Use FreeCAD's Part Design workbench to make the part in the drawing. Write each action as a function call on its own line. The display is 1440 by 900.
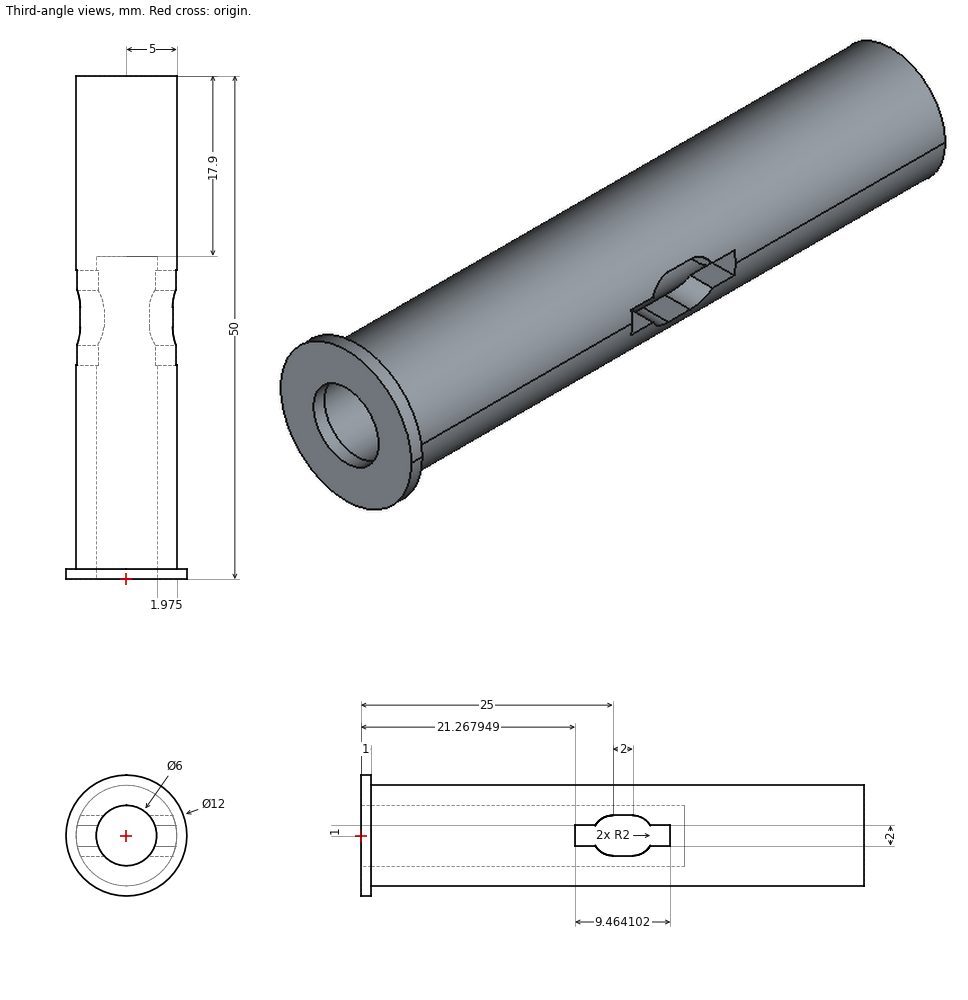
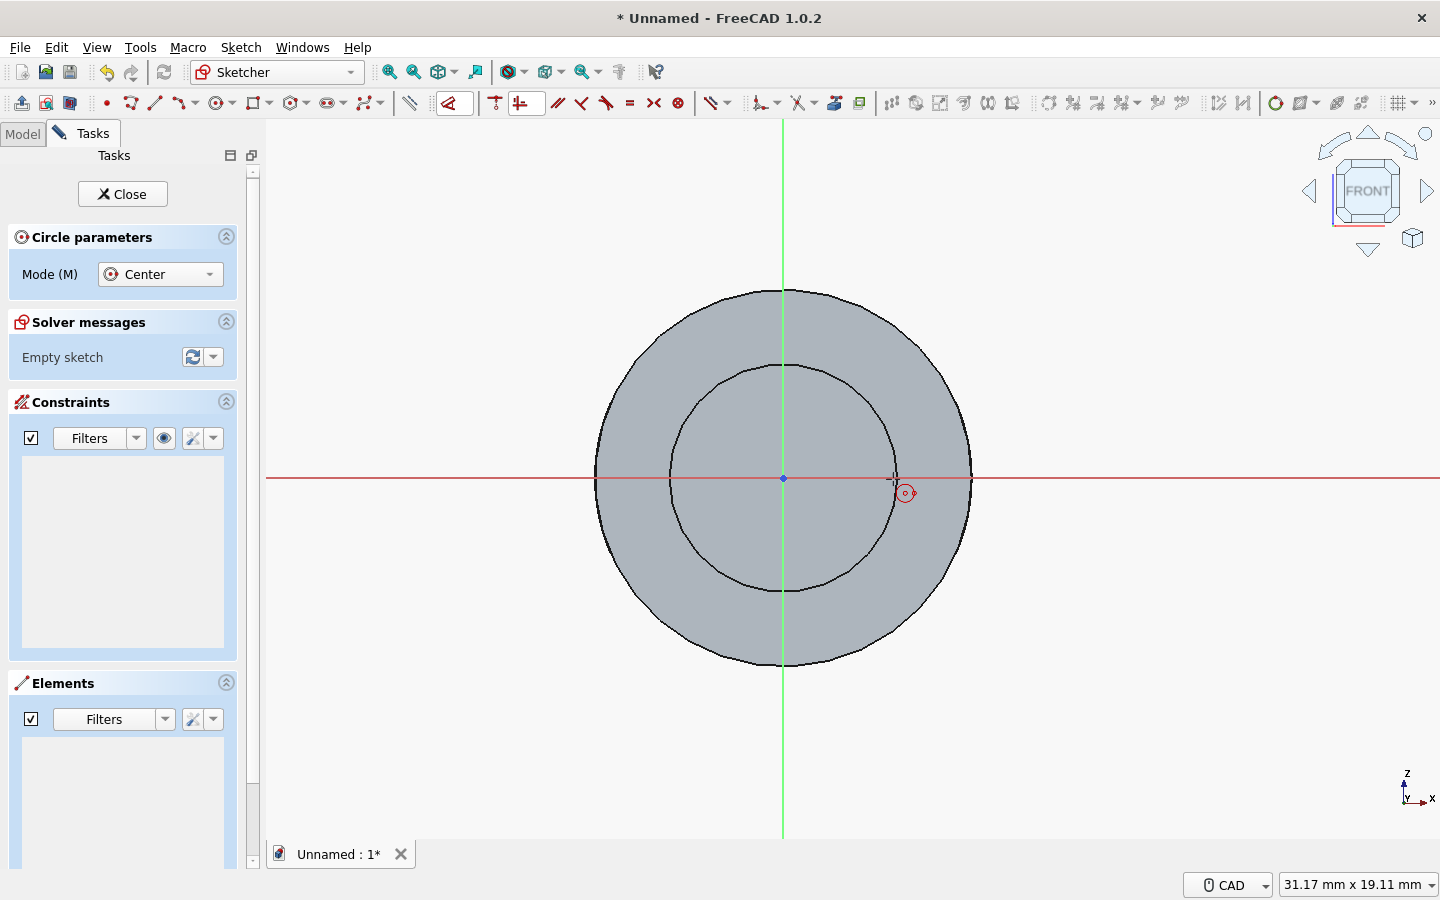
click(783, 478)
move(943, 318)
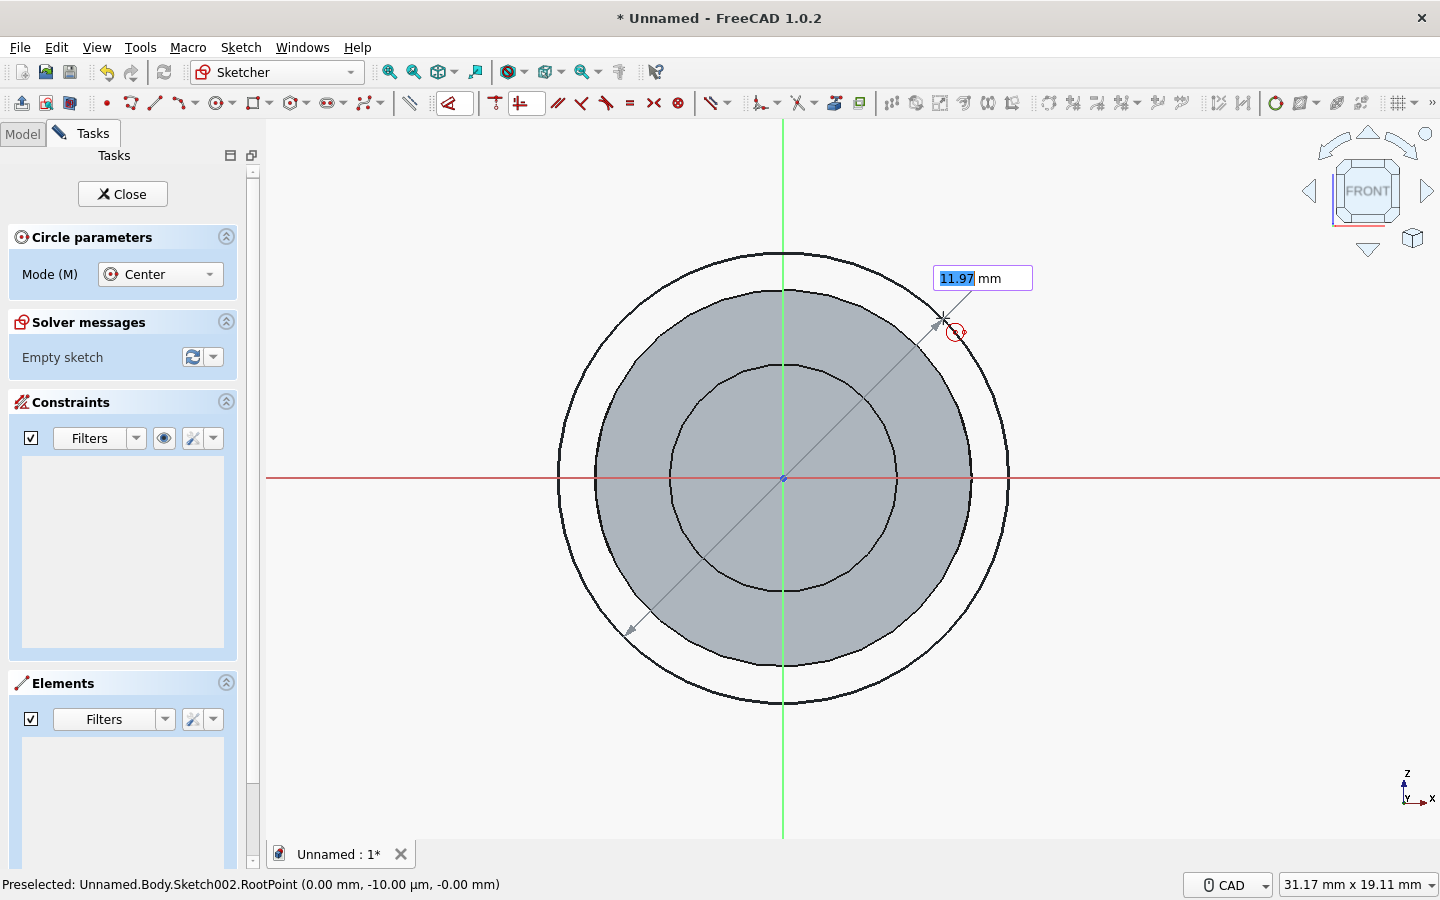
text(12)
key(Return)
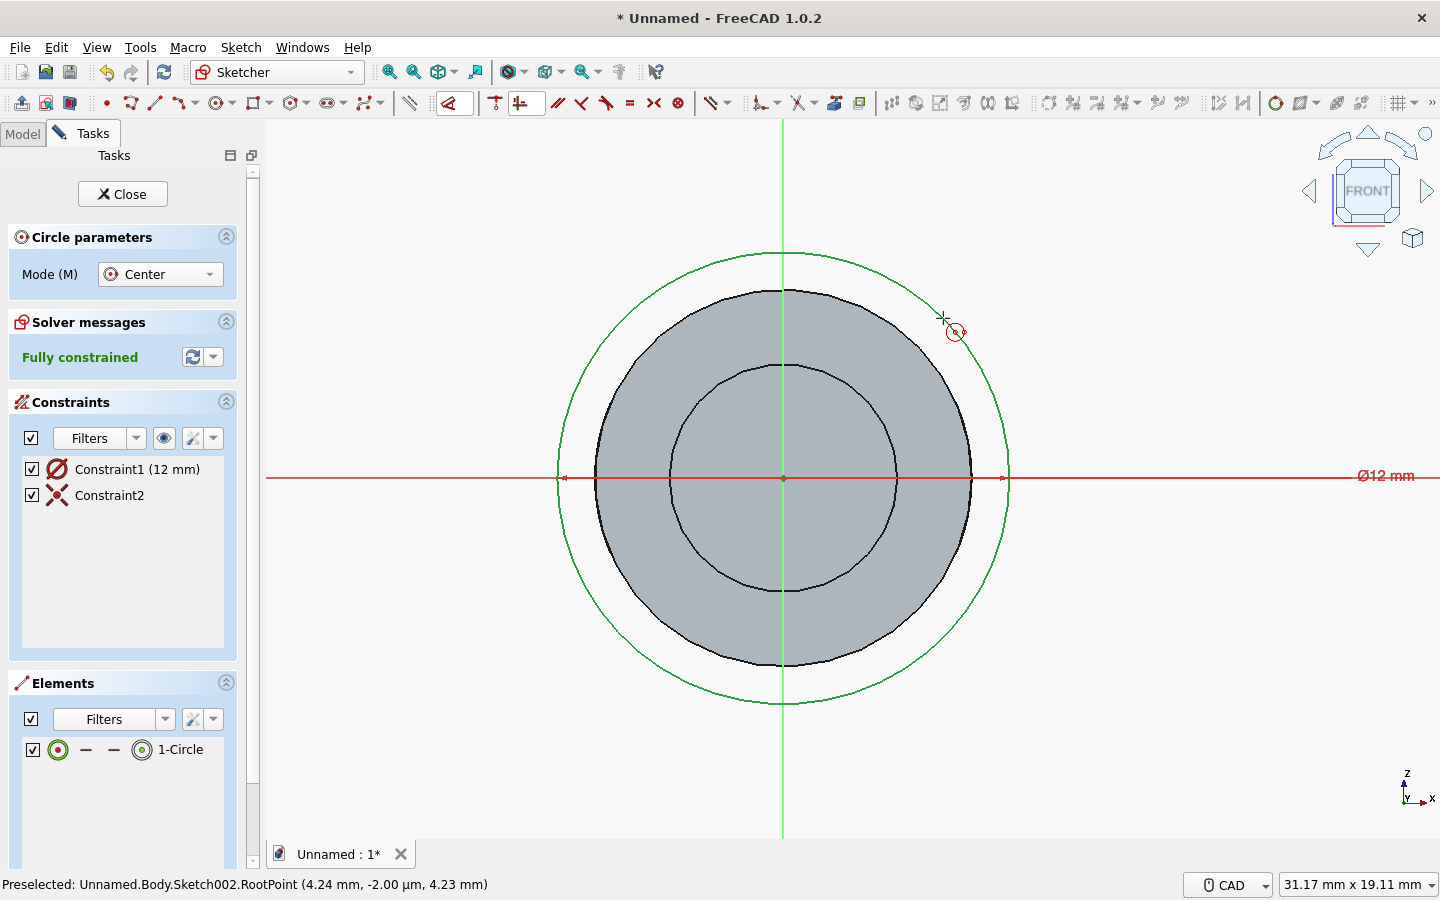
click(783, 478)
move(863, 398)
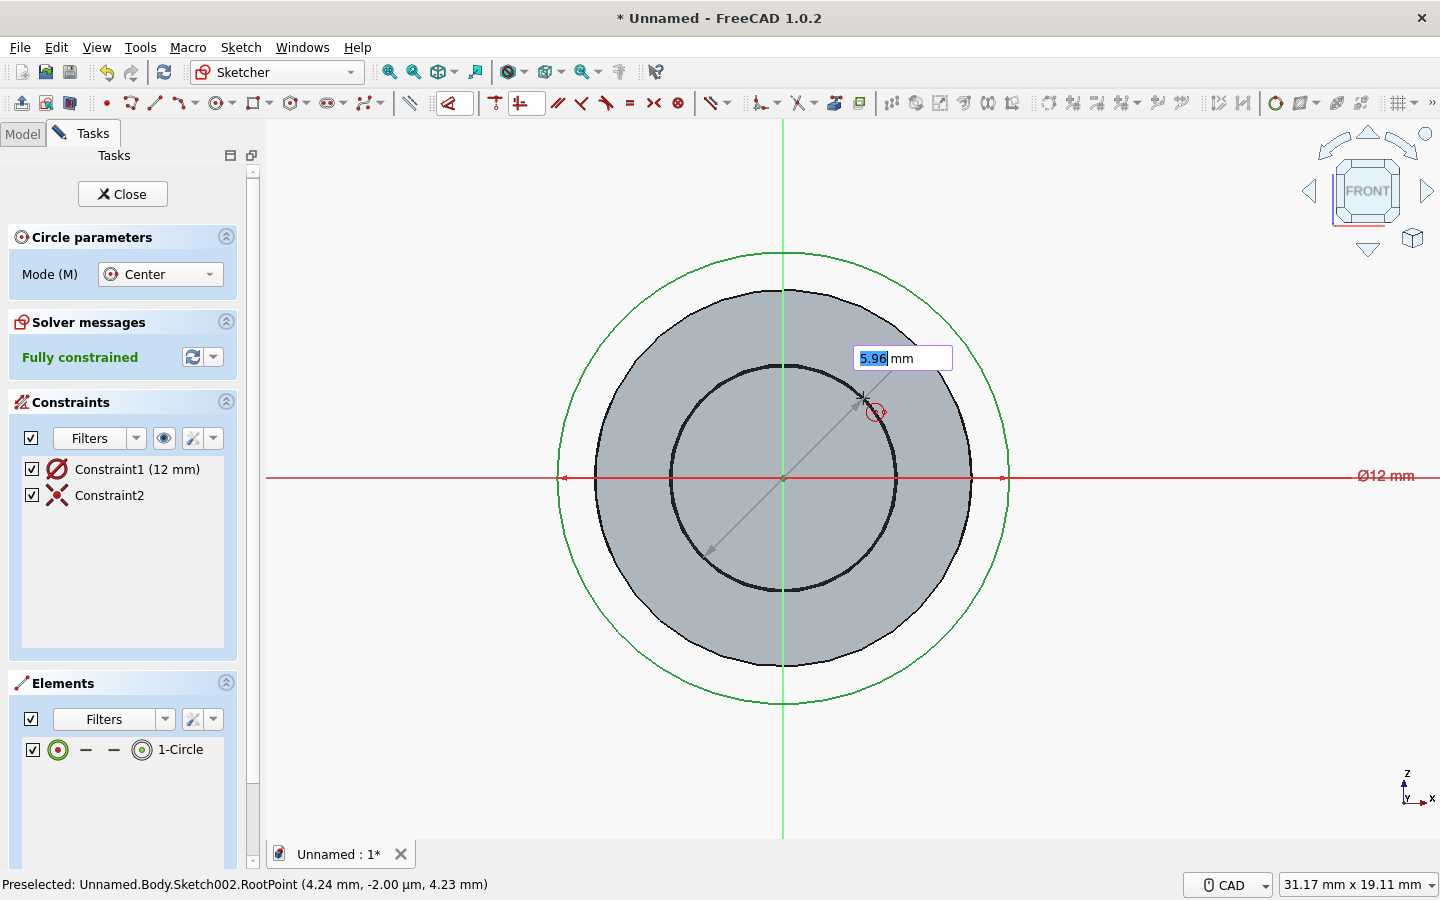
text(6)
key(Return)
key(Escape)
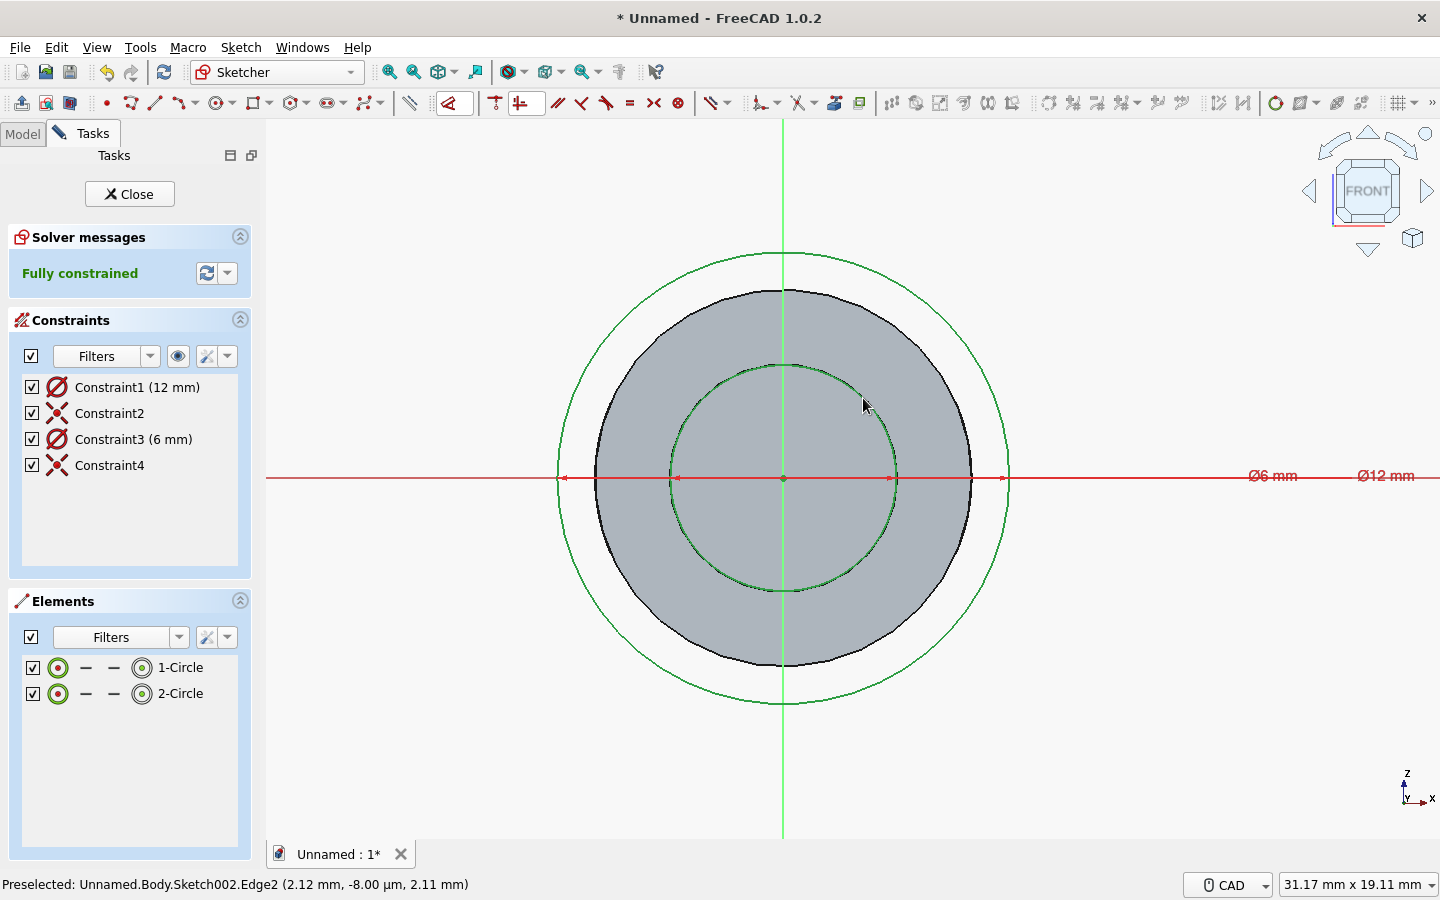
click(130, 194)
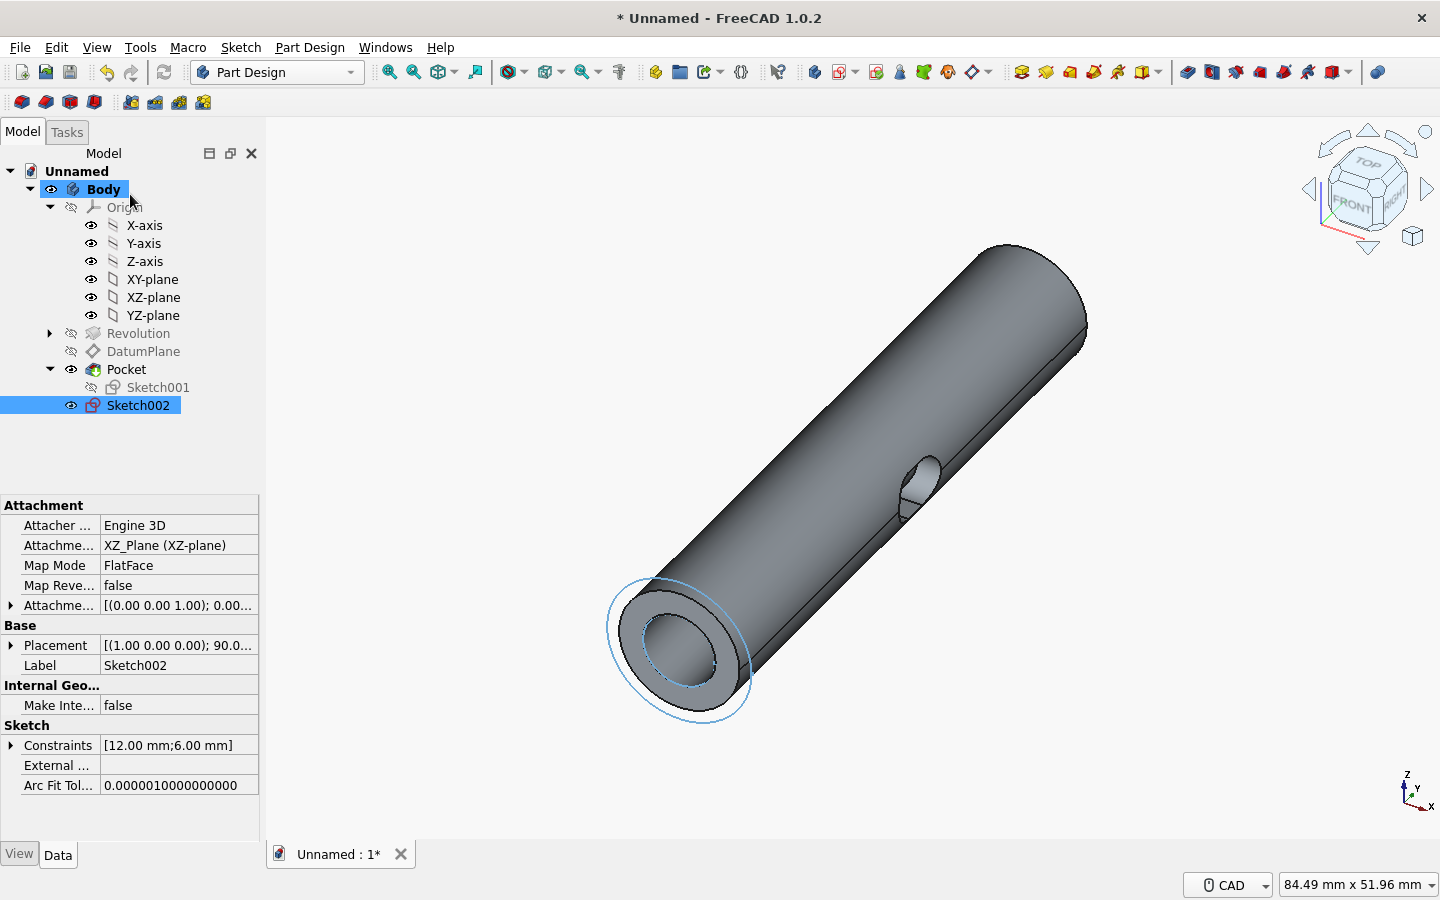
click(1022, 72)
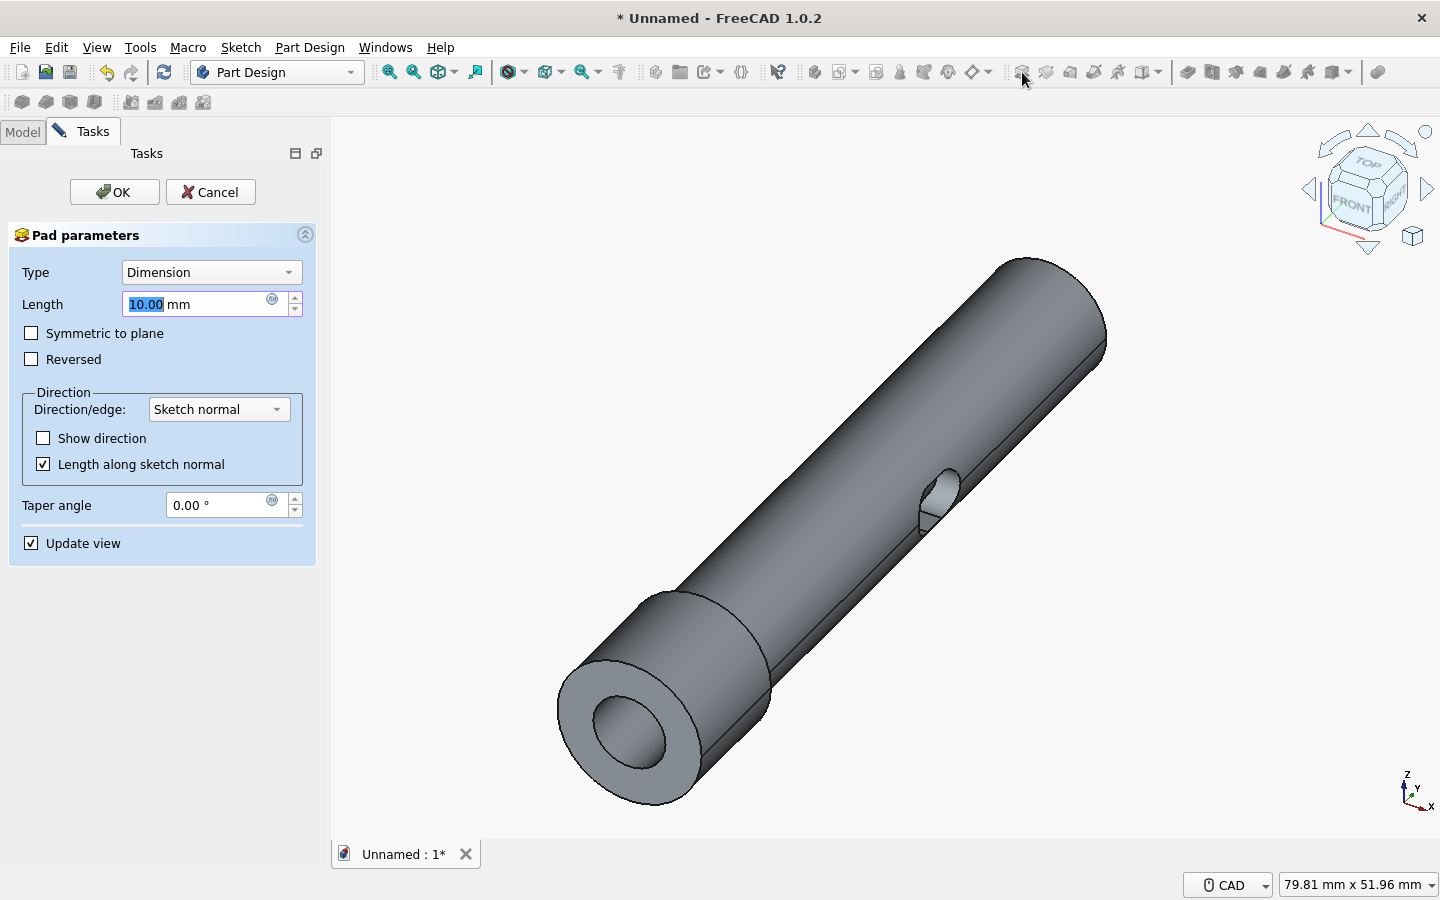
text(1)
key(Tab)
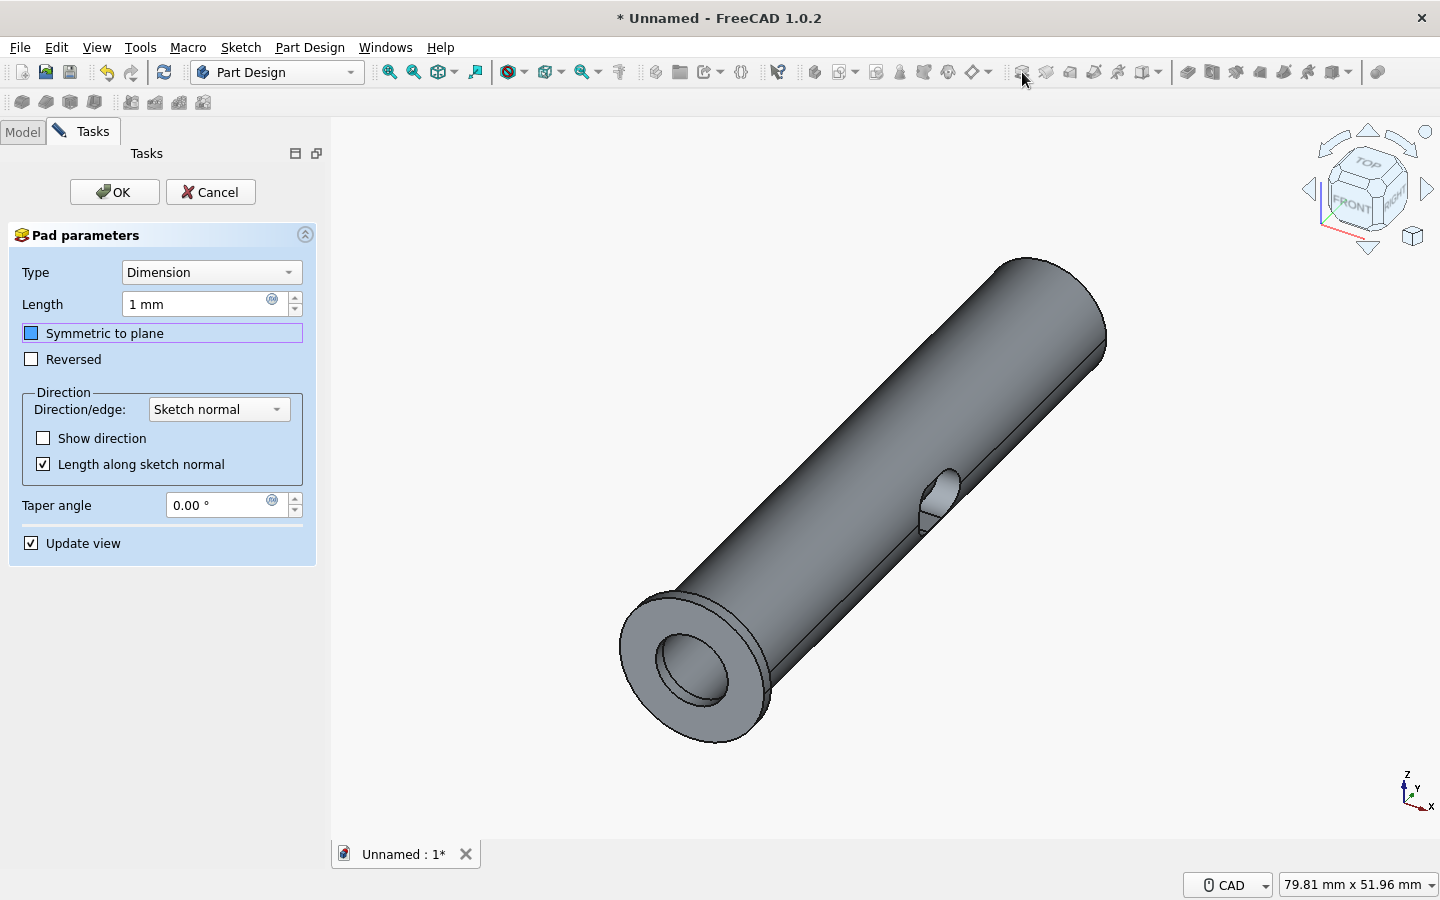
click(30, 359)